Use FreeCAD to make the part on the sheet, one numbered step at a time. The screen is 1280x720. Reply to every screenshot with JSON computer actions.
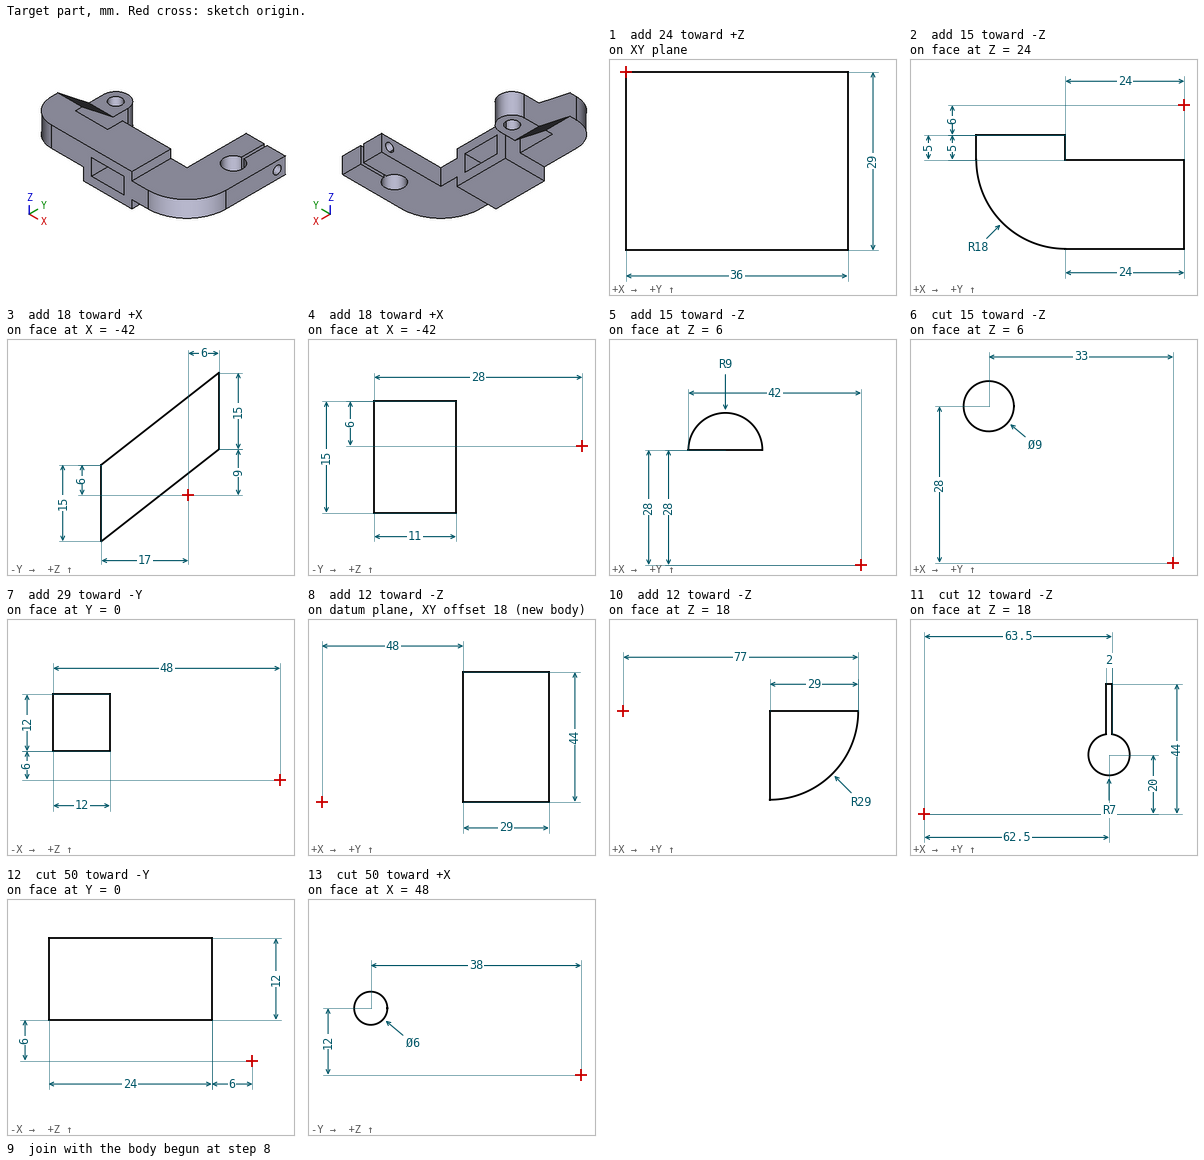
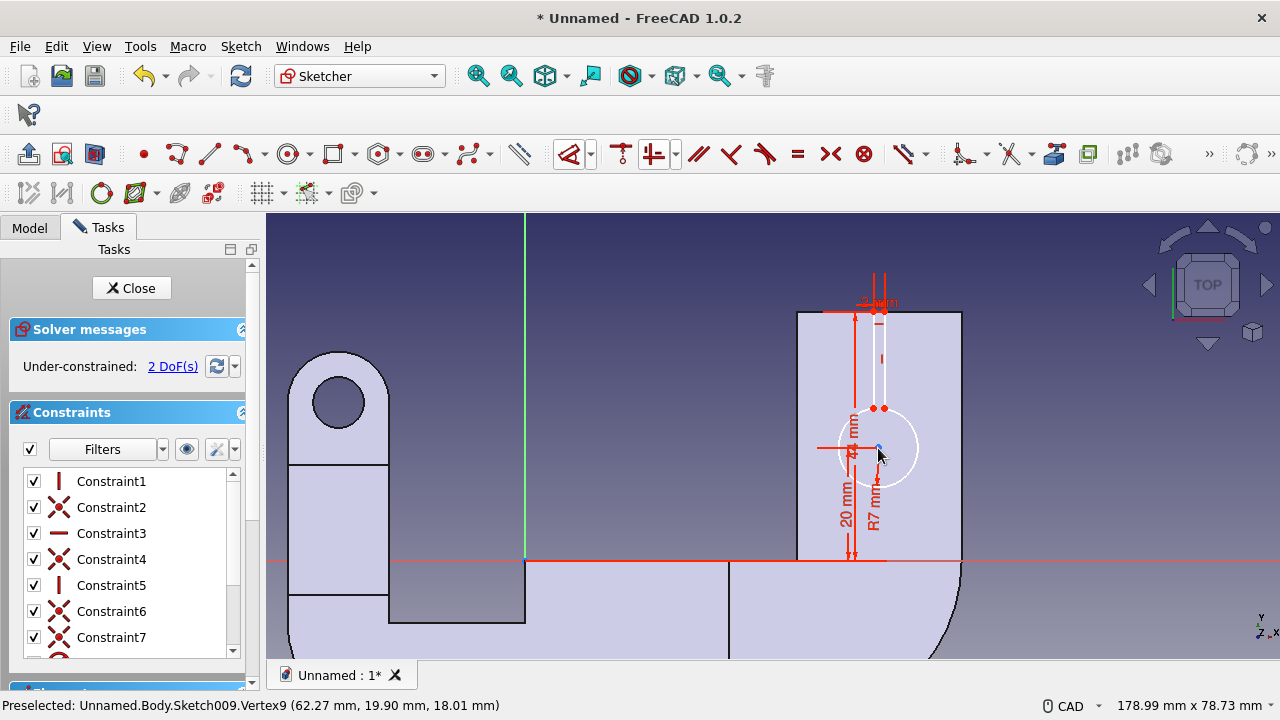
{"action": "left_click", "coordinate": [885, 409]}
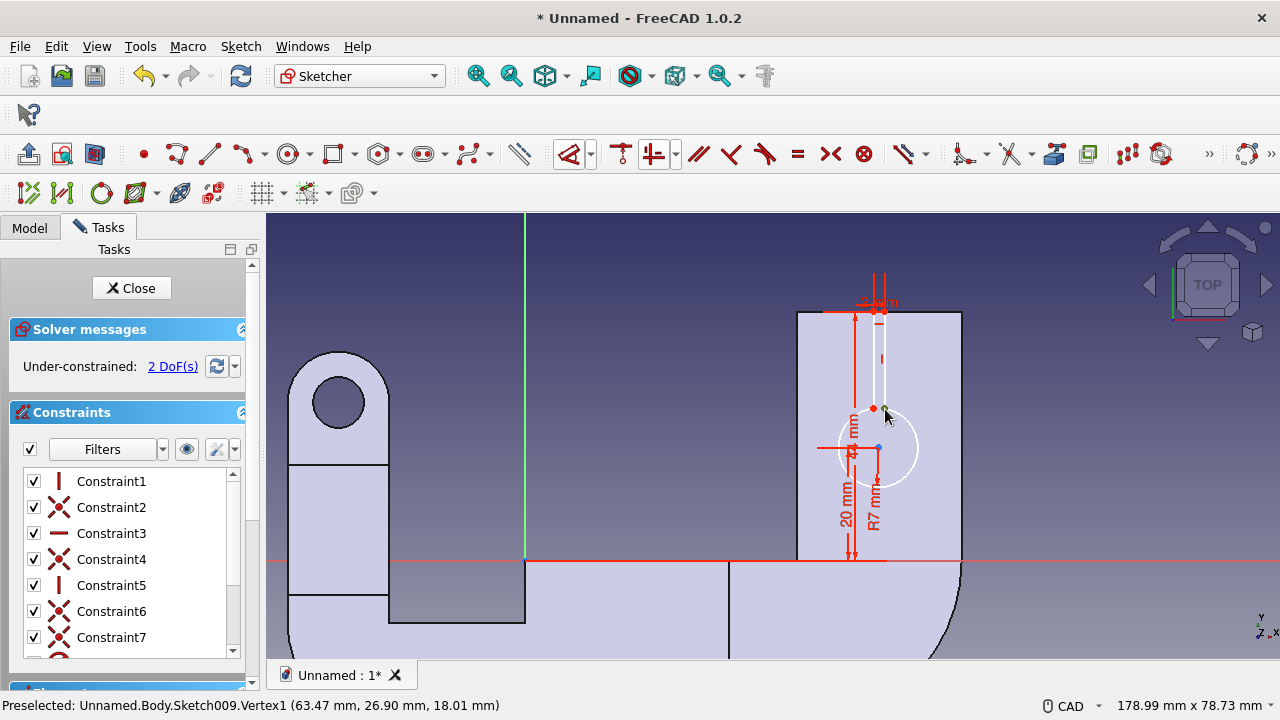
{"action": "left_click", "coordinate": [590, 154]}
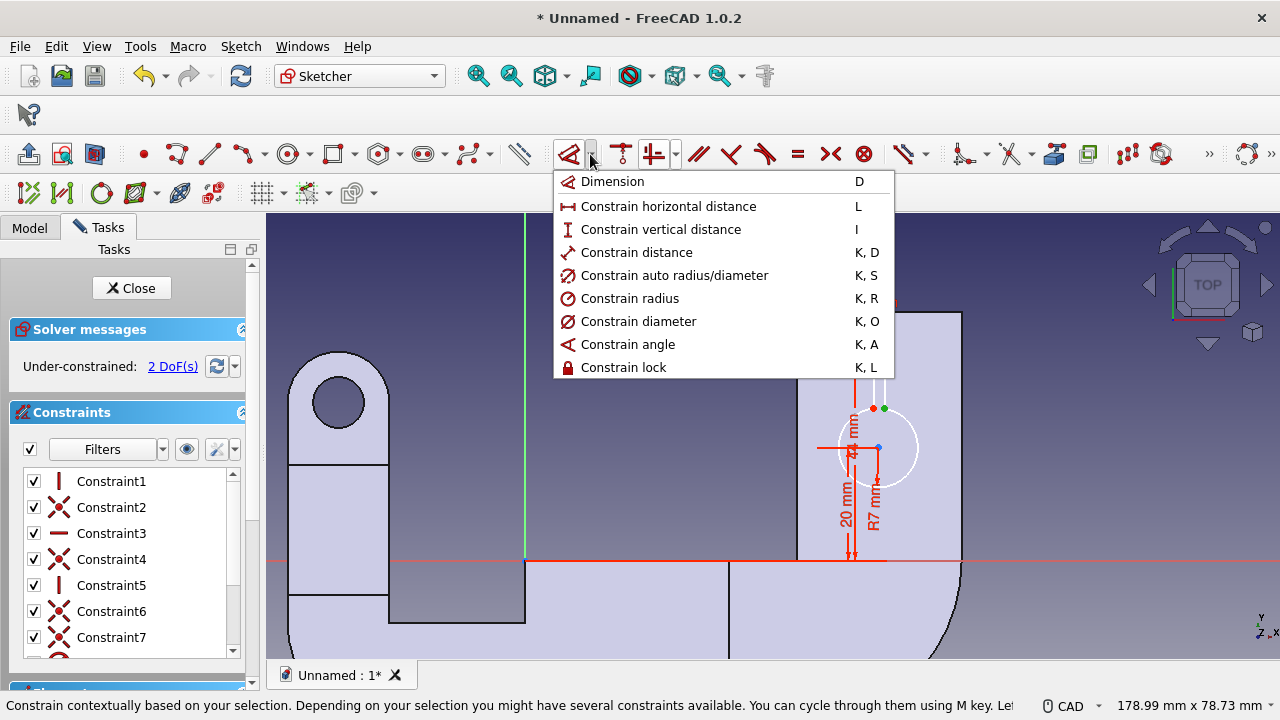
{"action": "left_click", "coordinate": [724, 206]}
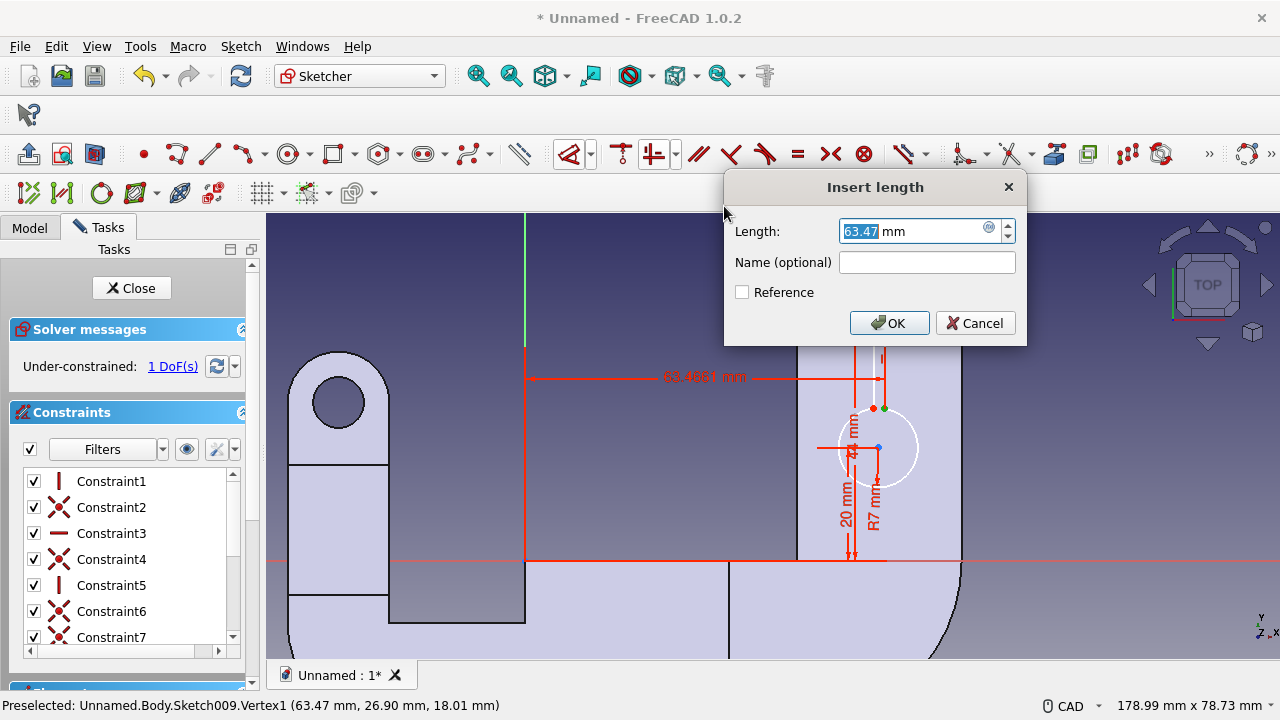
{"action": "type", "text": "63.5"}
{"action": "key", "text": "Return"}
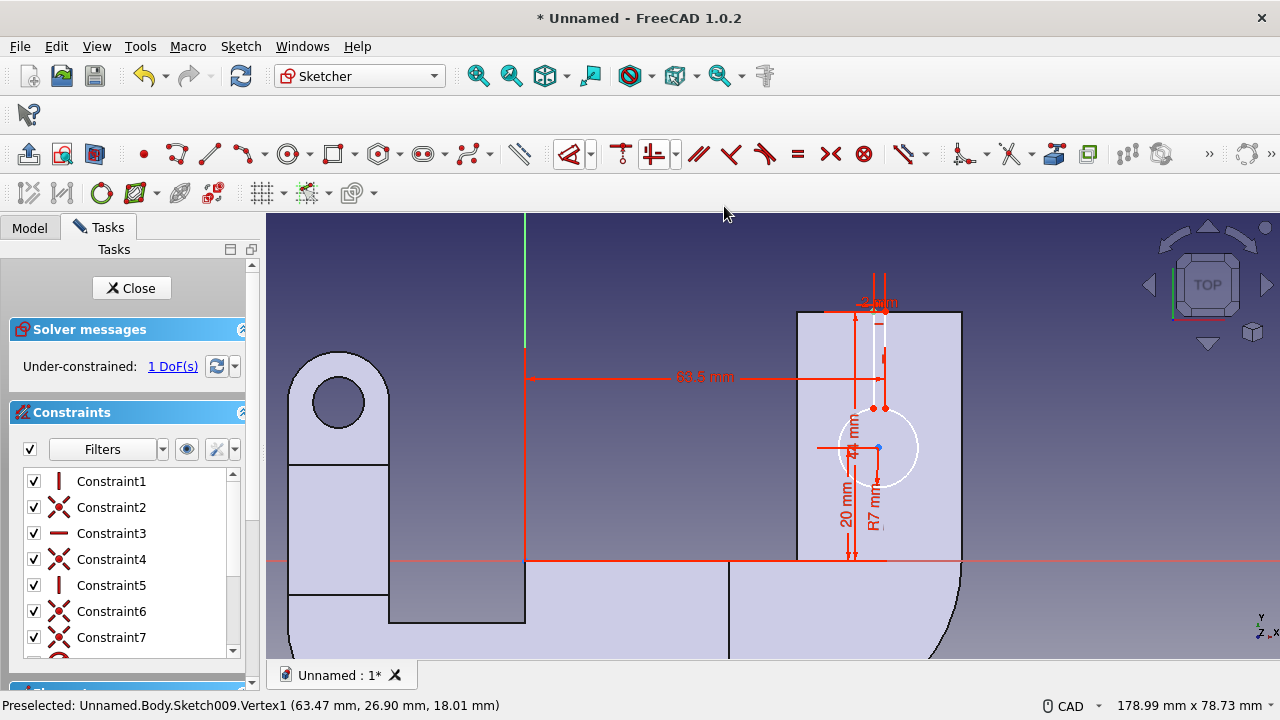
{"action": "left_click", "coordinate": [878, 448]}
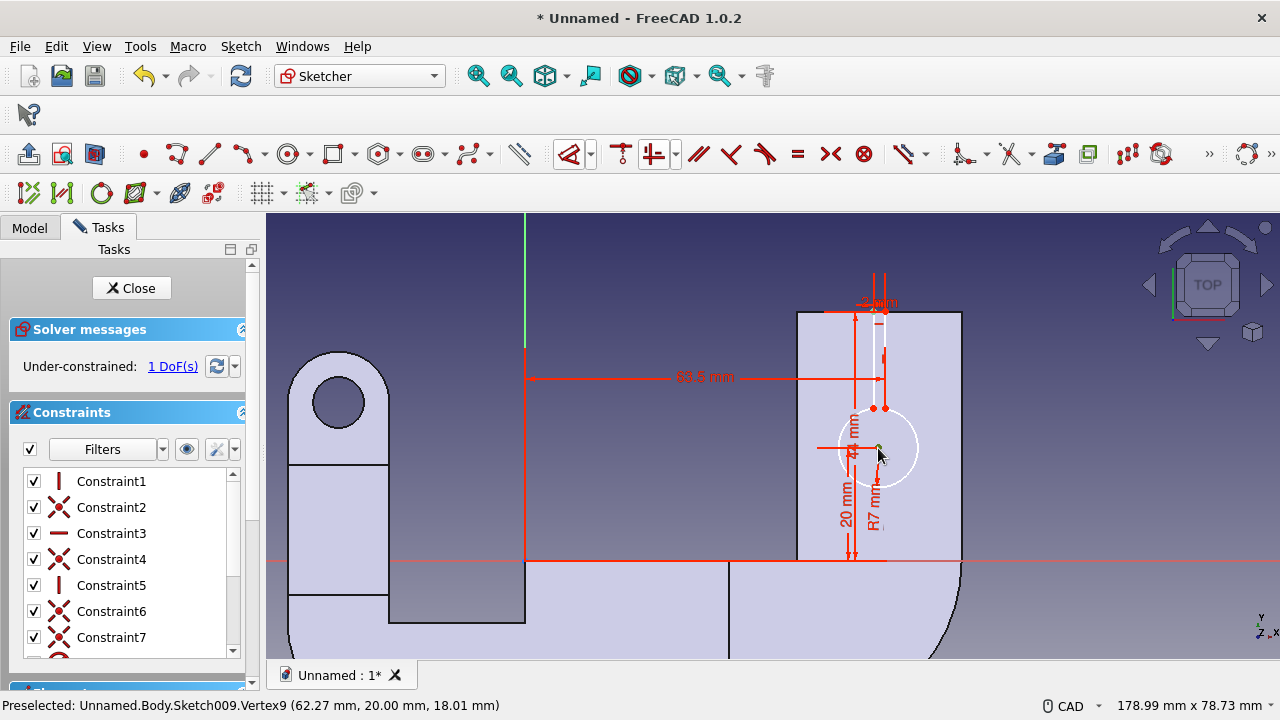
{"action": "left_click", "coordinate": [590, 154]}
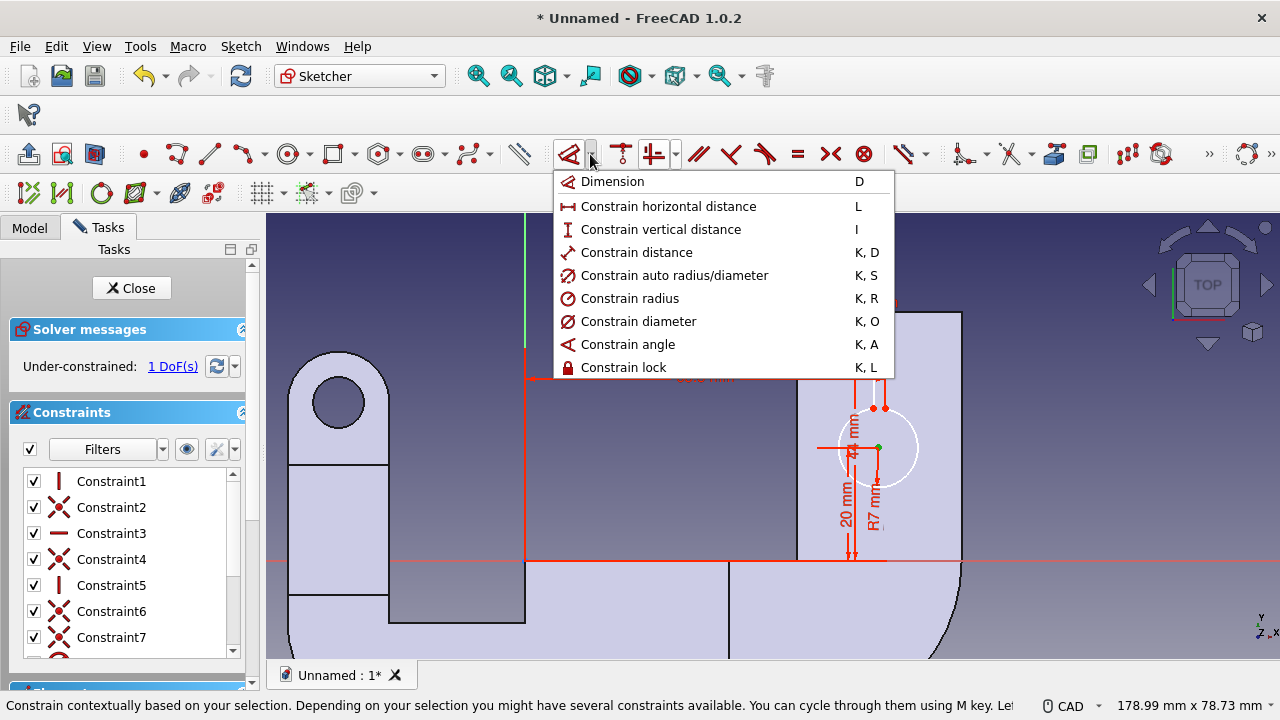
{"action": "left_click", "coordinate": [724, 206]}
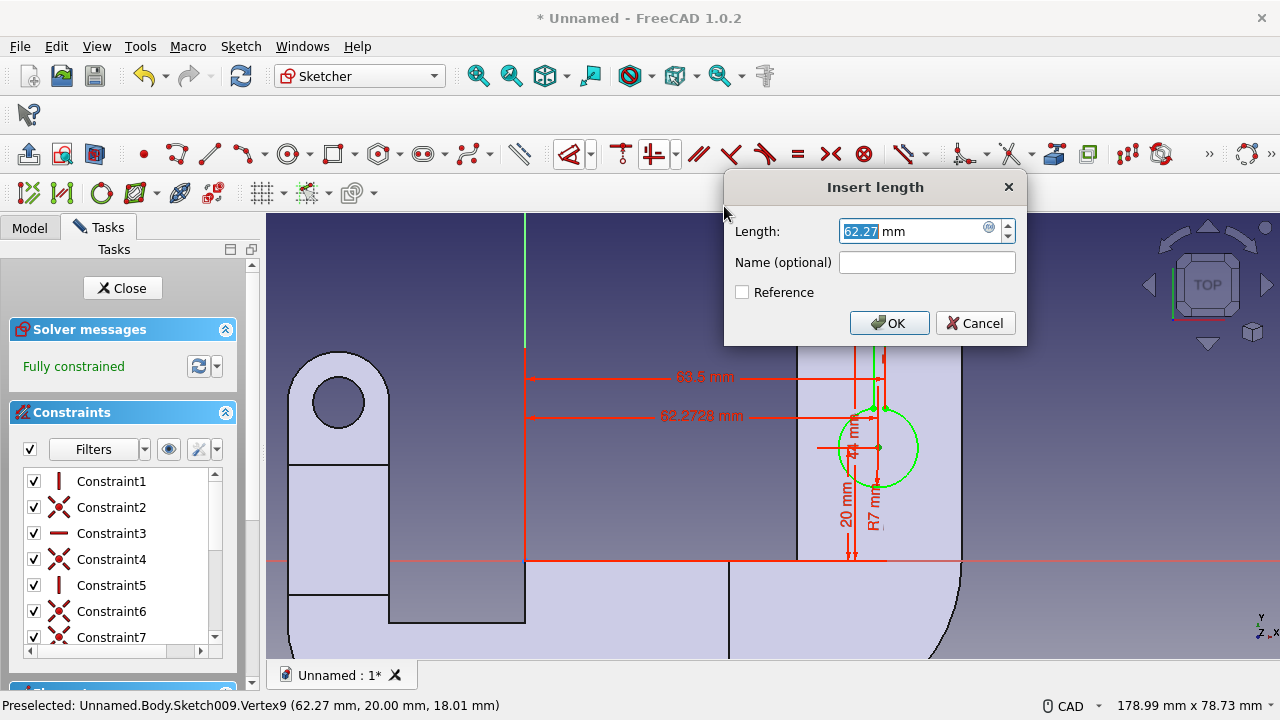
{"action": "type", "text": "62.5"}
{"action": "key", "text": "Return"}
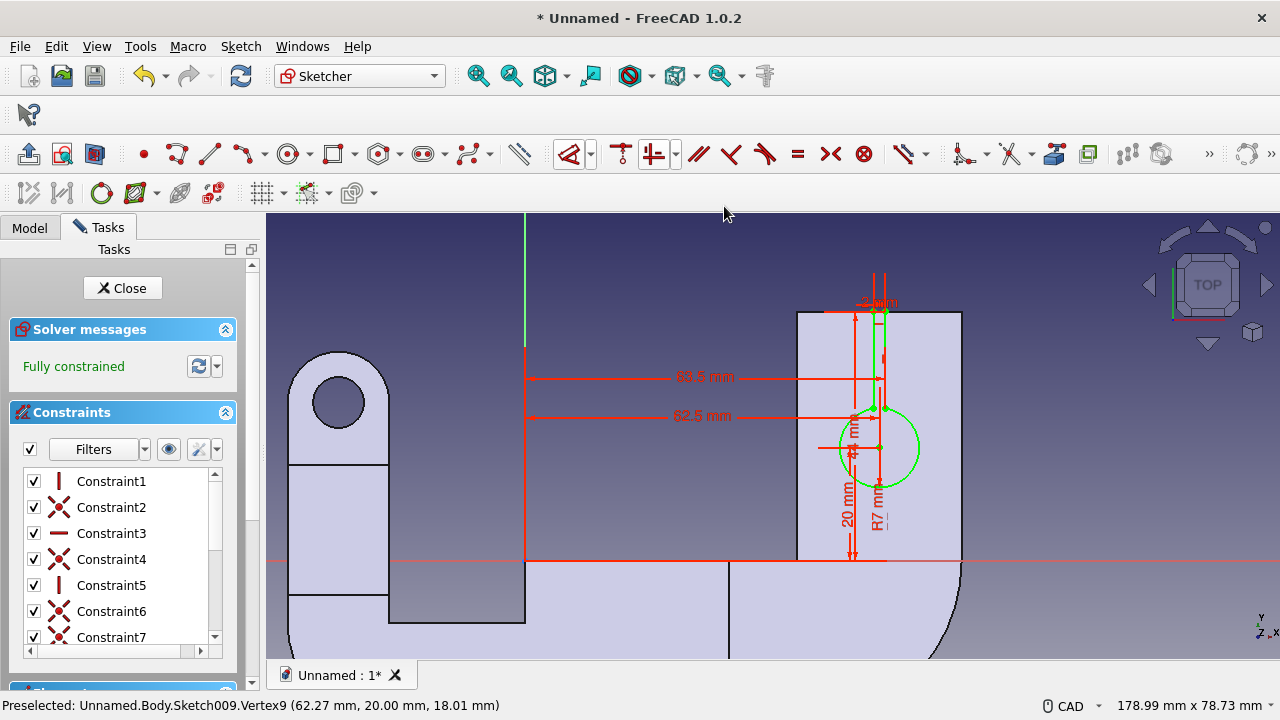
{"action": "left_click", "coordinate": [123, 288]}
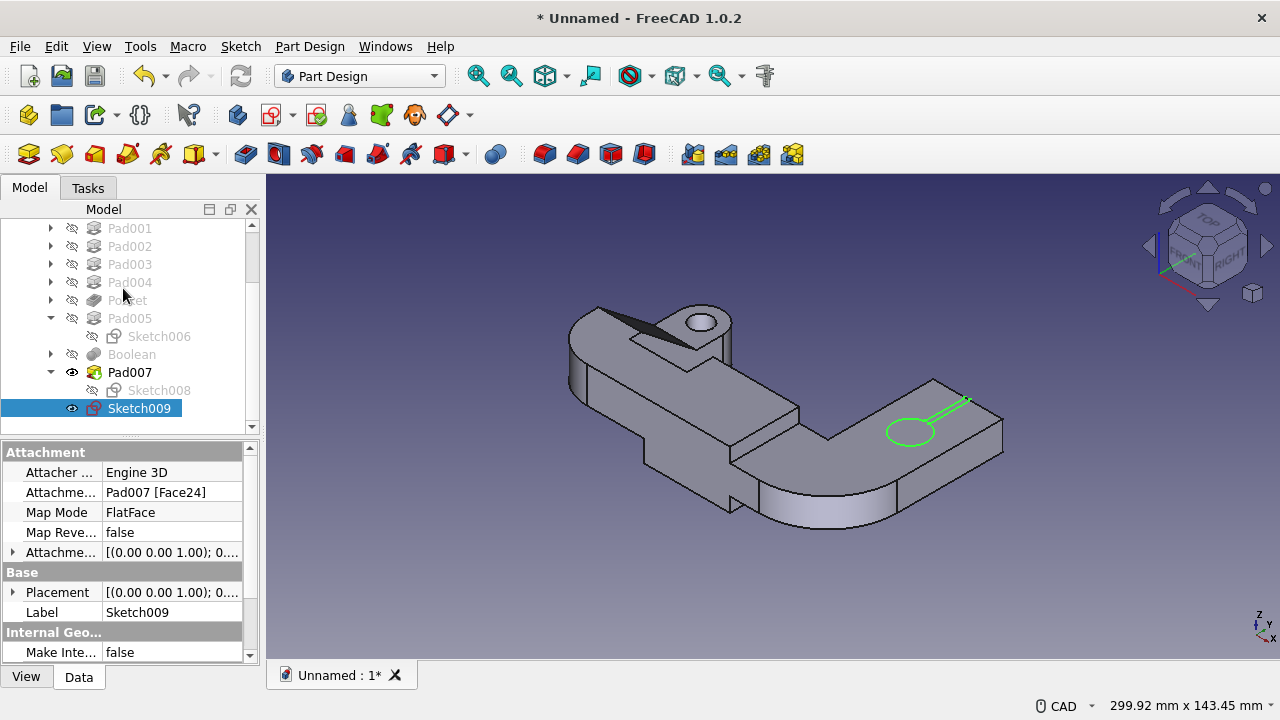
{"action": "left_click", "coordinate": [246, 154]}